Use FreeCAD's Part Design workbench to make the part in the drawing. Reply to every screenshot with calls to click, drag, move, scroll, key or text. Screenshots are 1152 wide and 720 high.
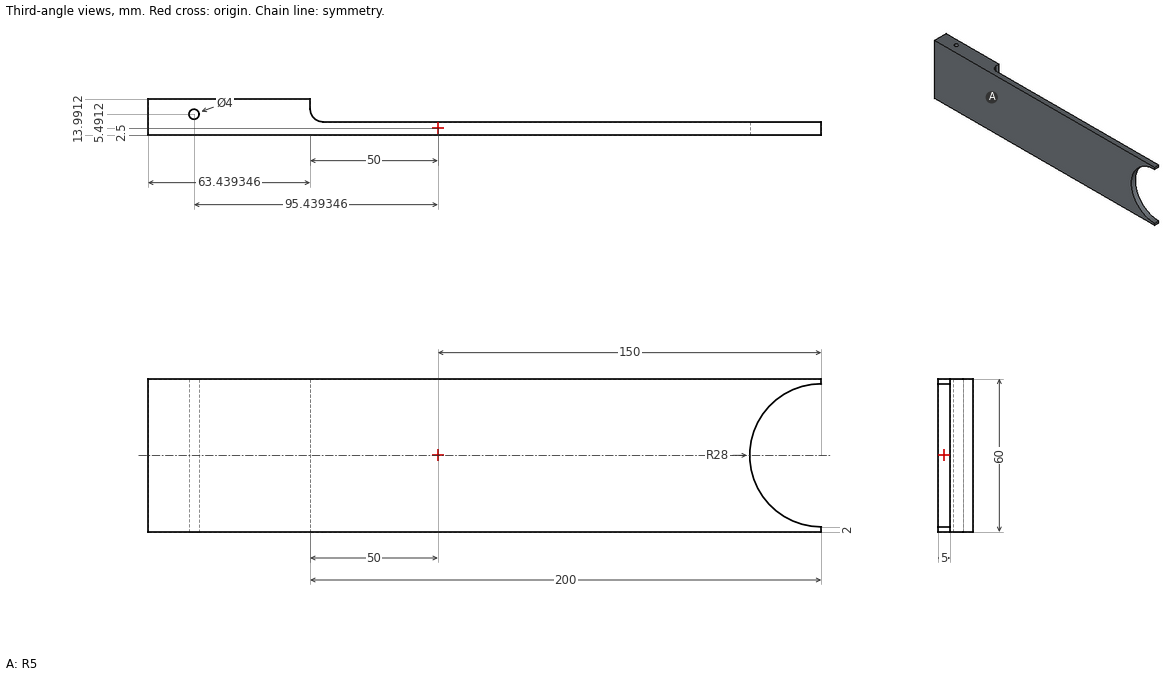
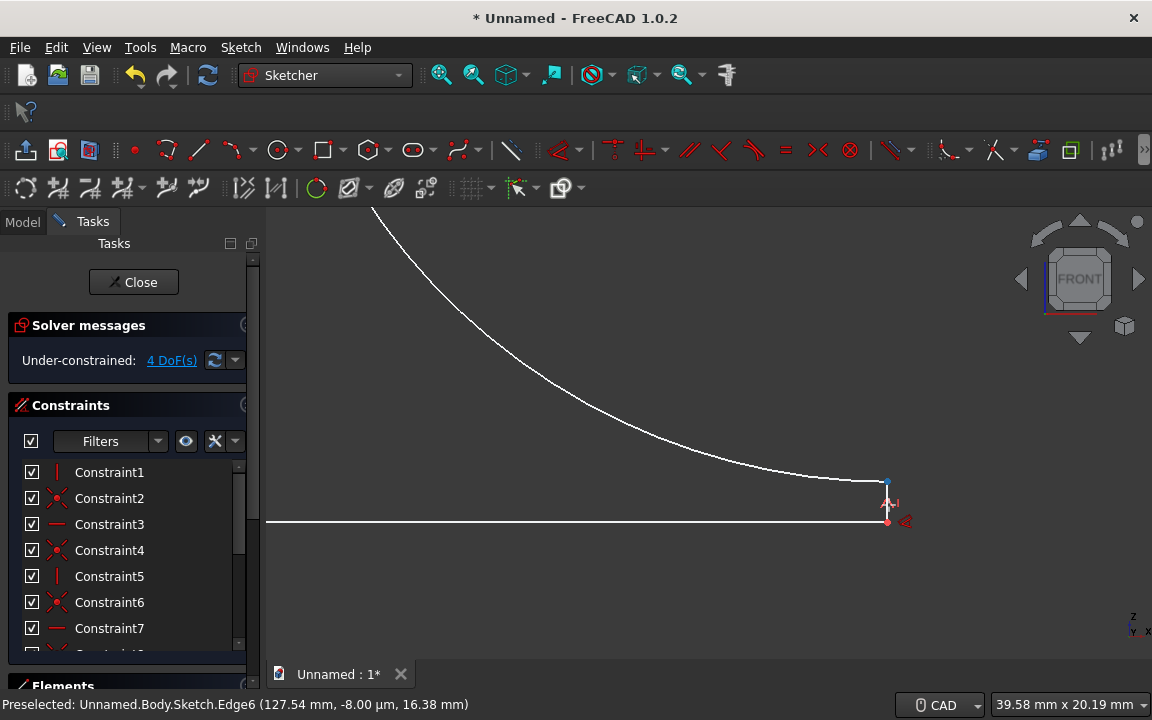
click(887, 502)
click(921, 502)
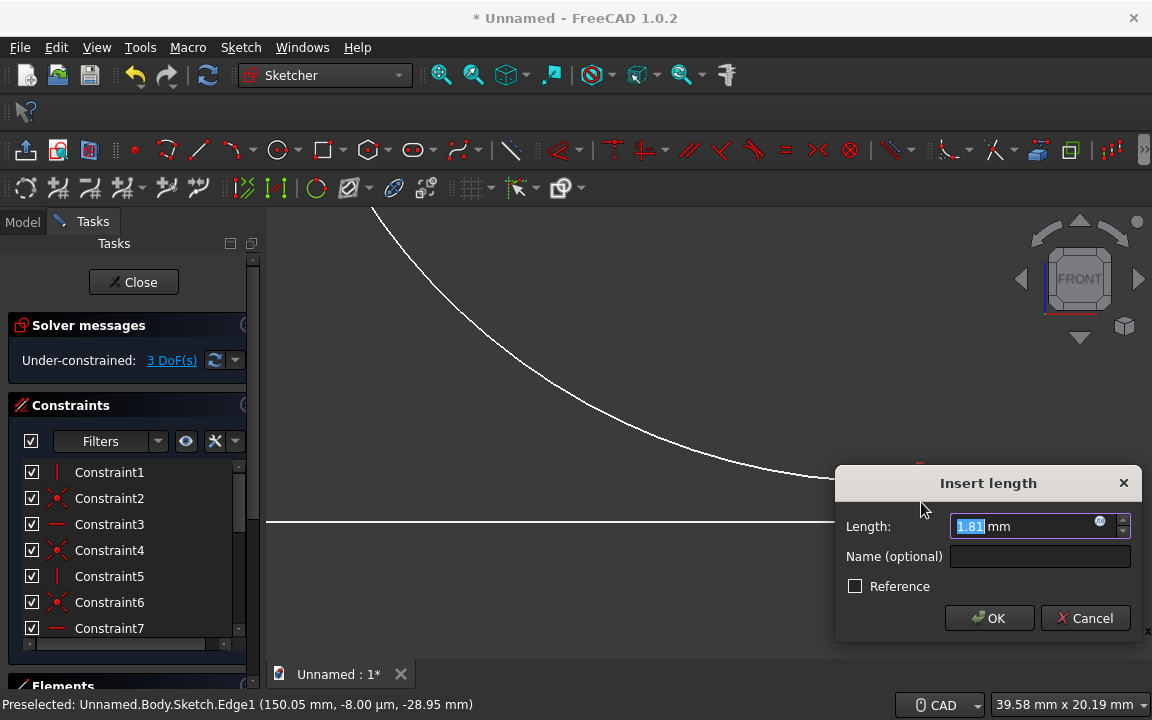
text(2)
key(Return)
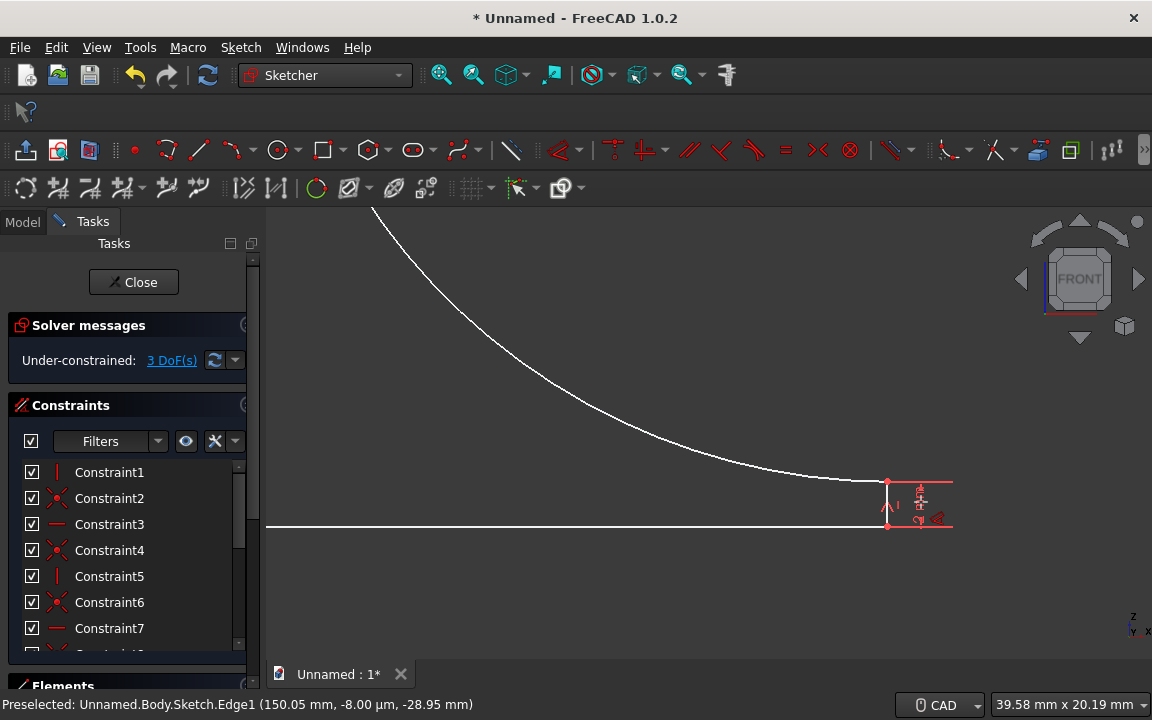
scroll(889, 505, down, 11)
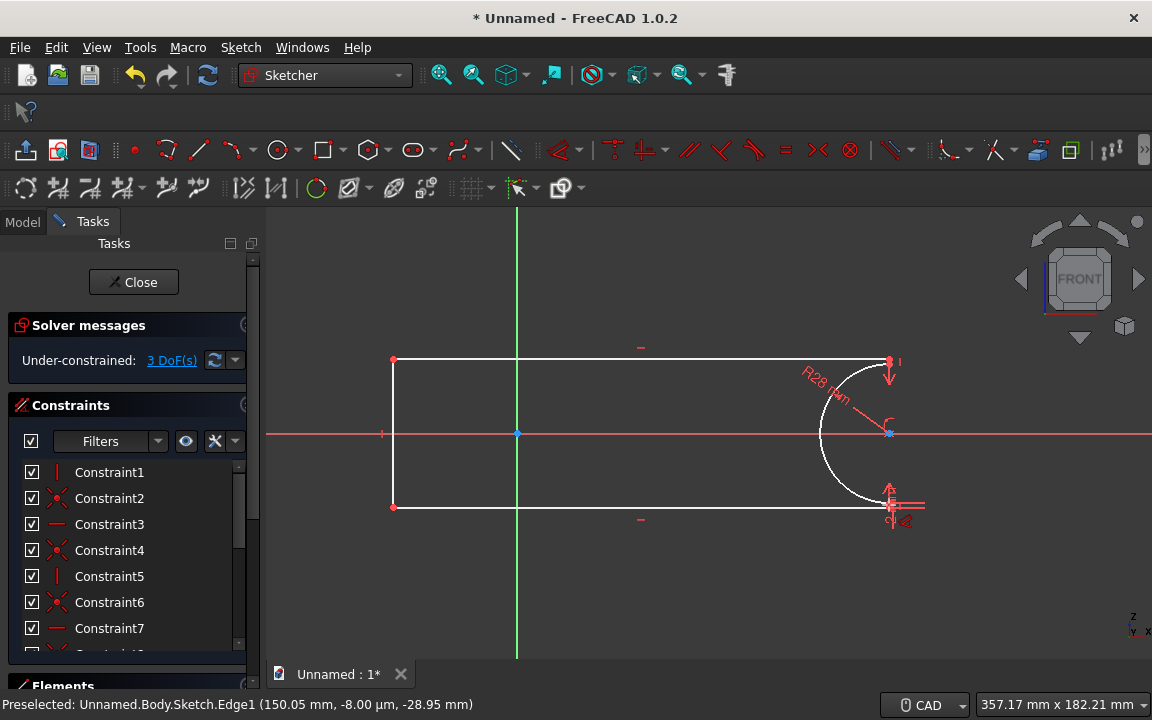
click(741, 508)
click(641, 542)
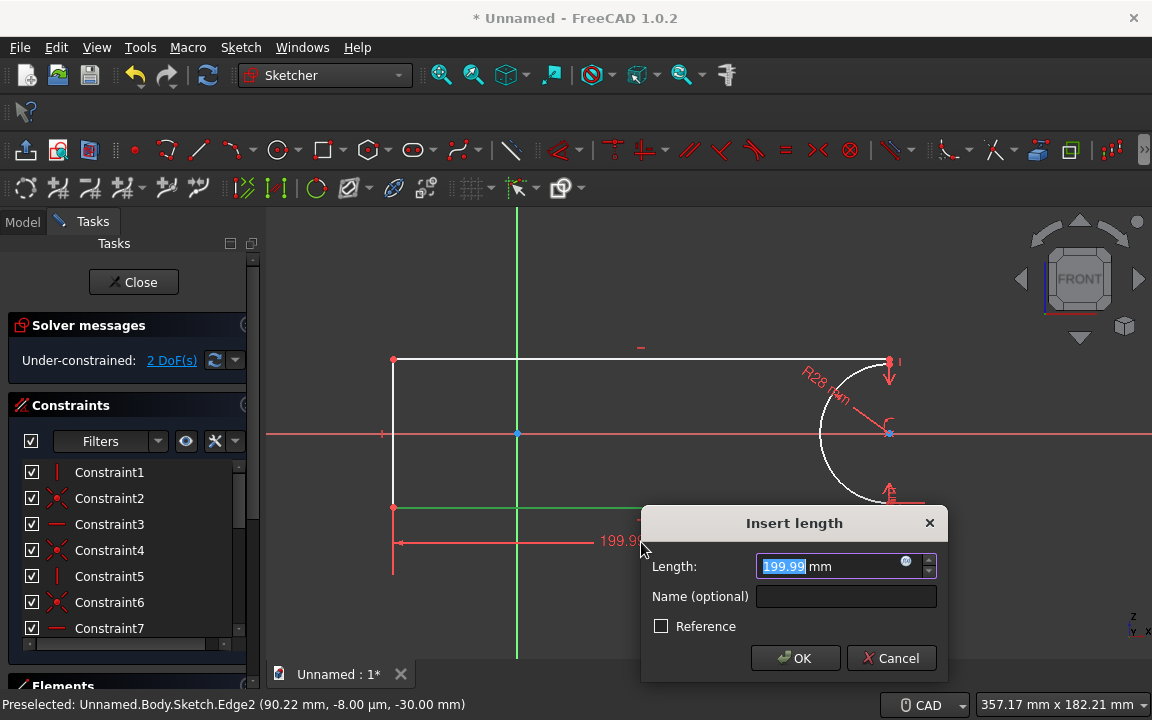
text(200)
key(Return)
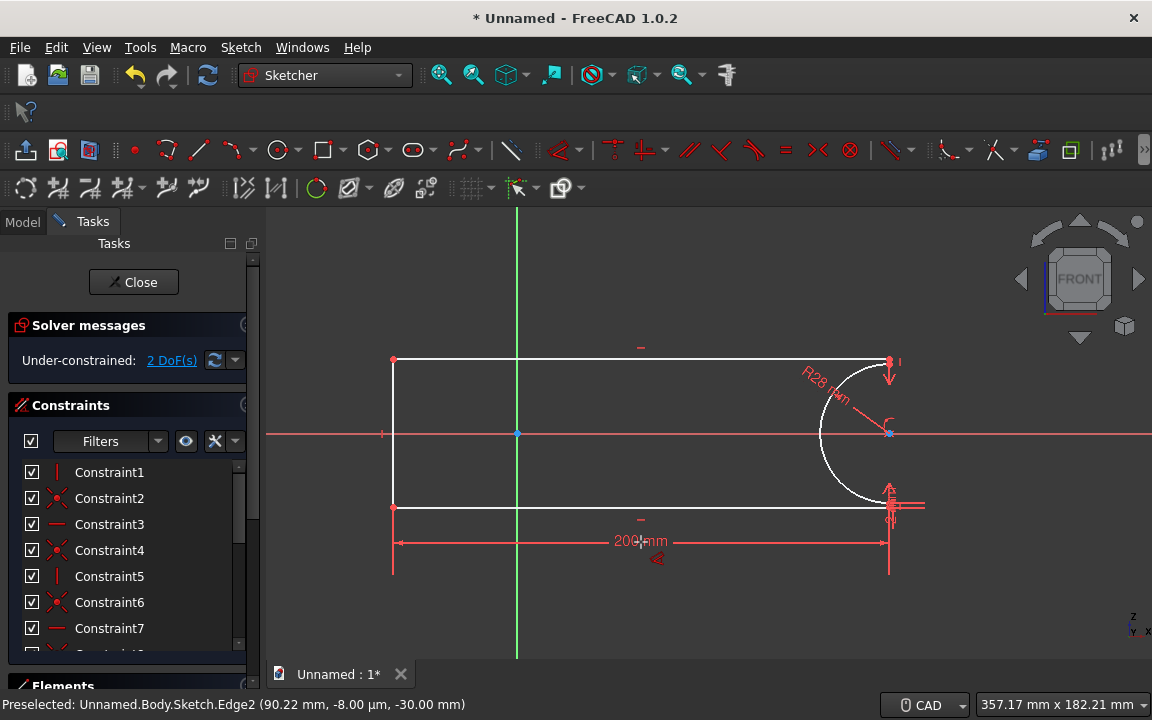
click(393, 508)
click(455, 542)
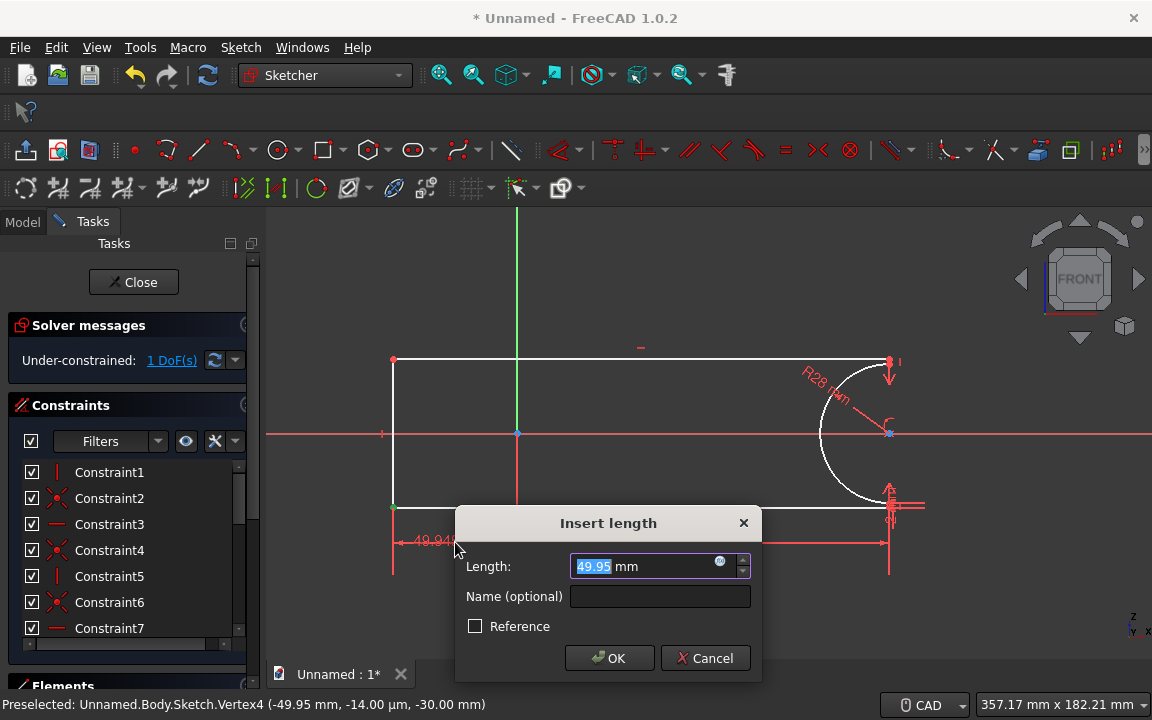
text(50)
key(Return)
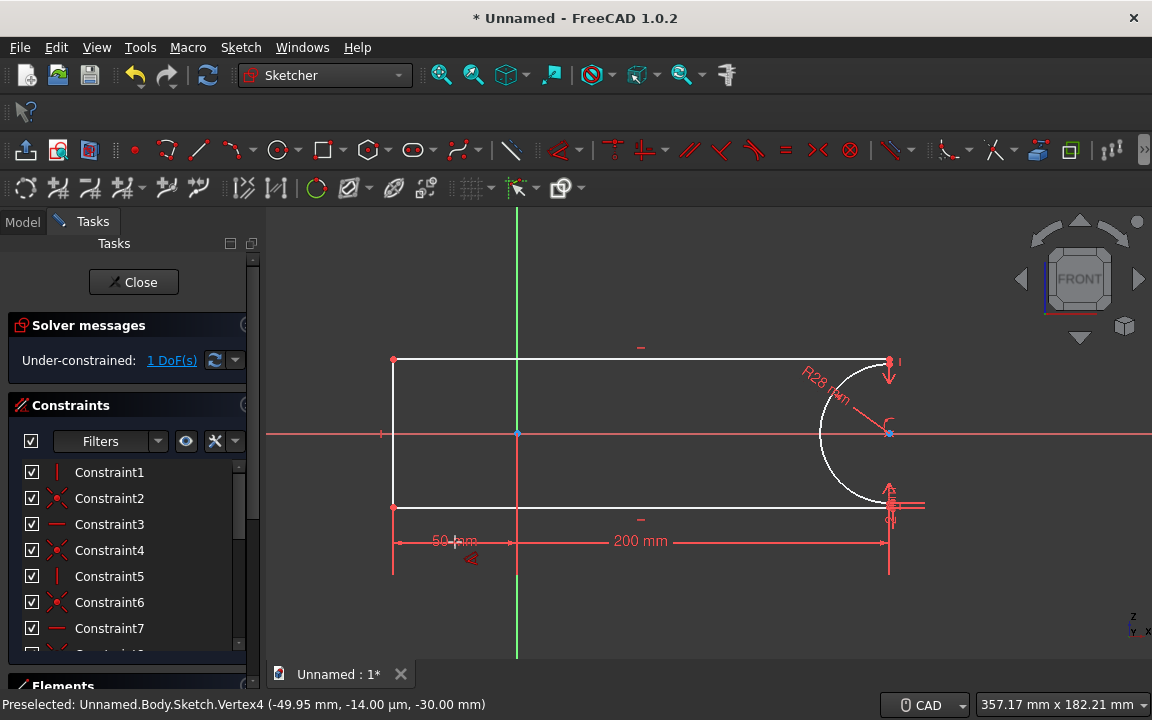
click(890, 434)
click(703, 468)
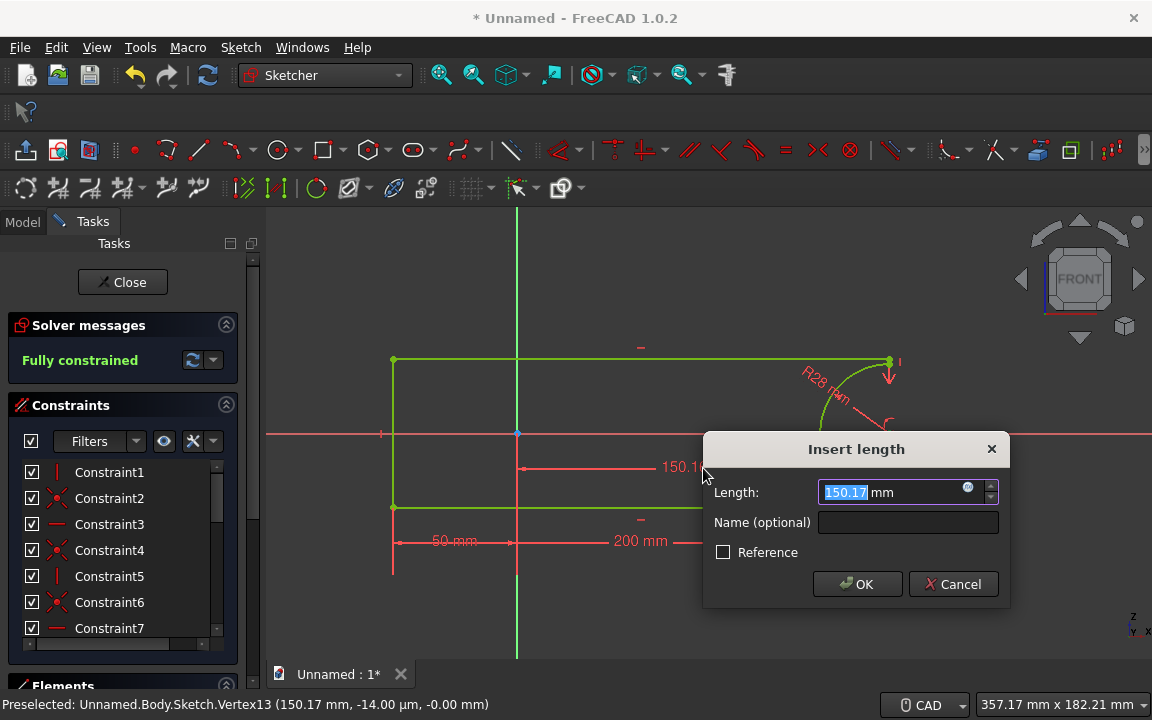
text(150)
key(Return)
key(Escape)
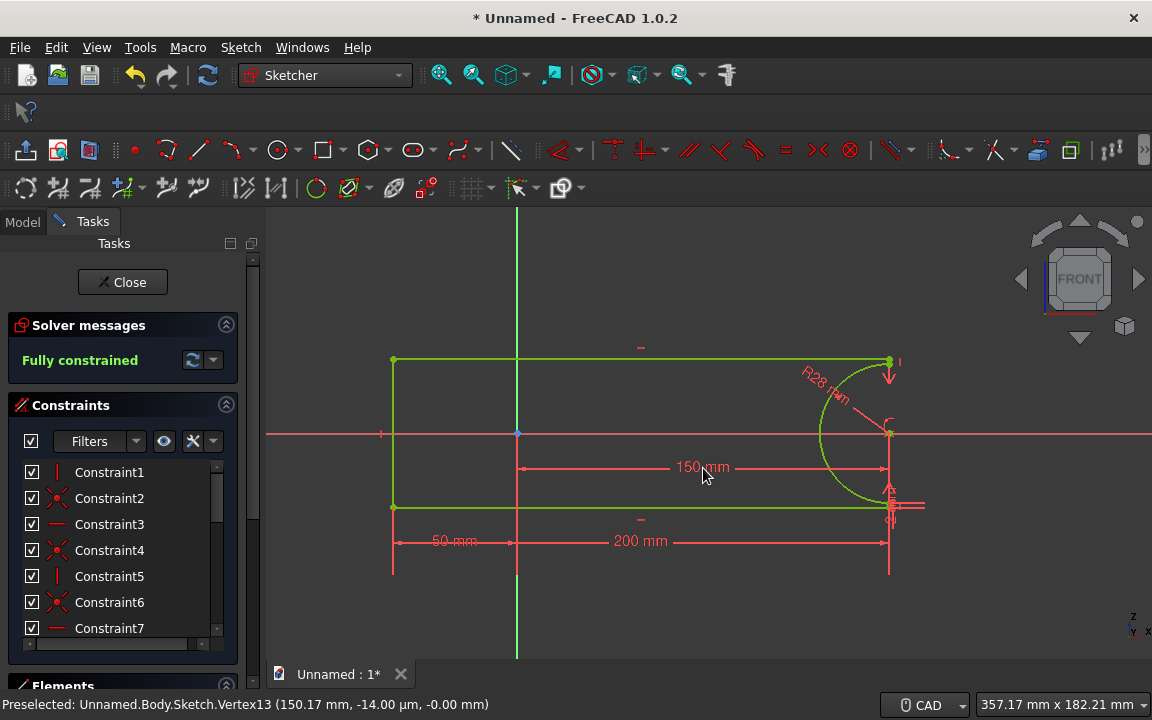
click(123, 282)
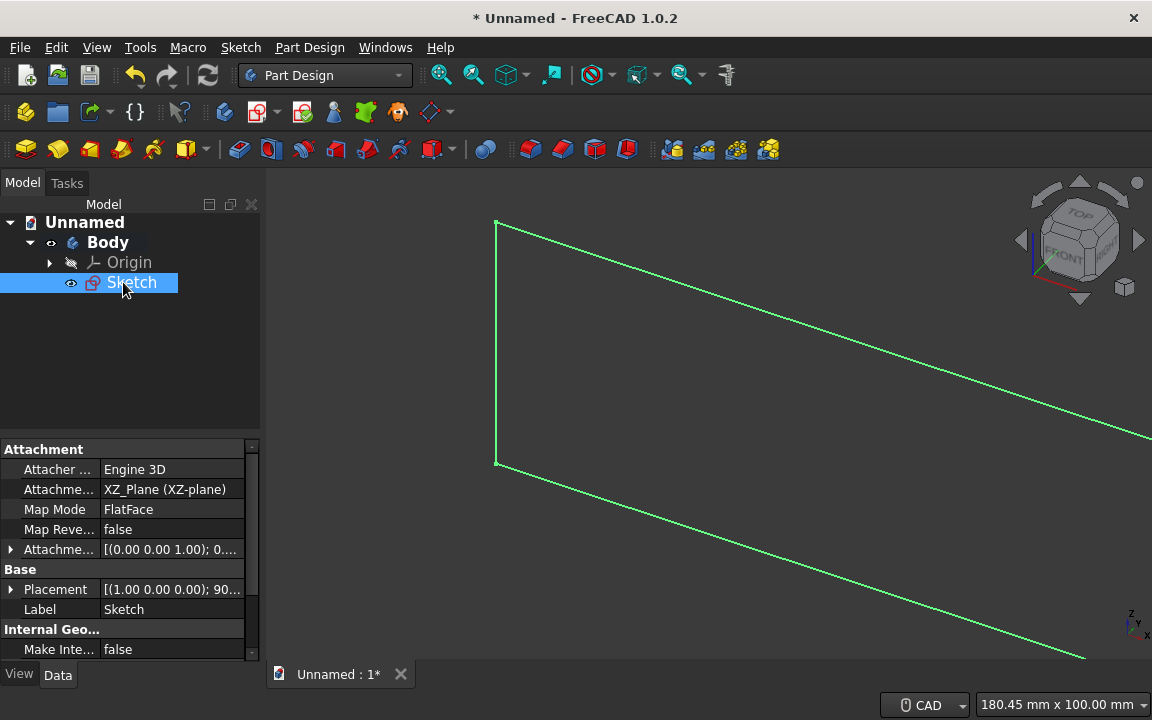
click(26, 150)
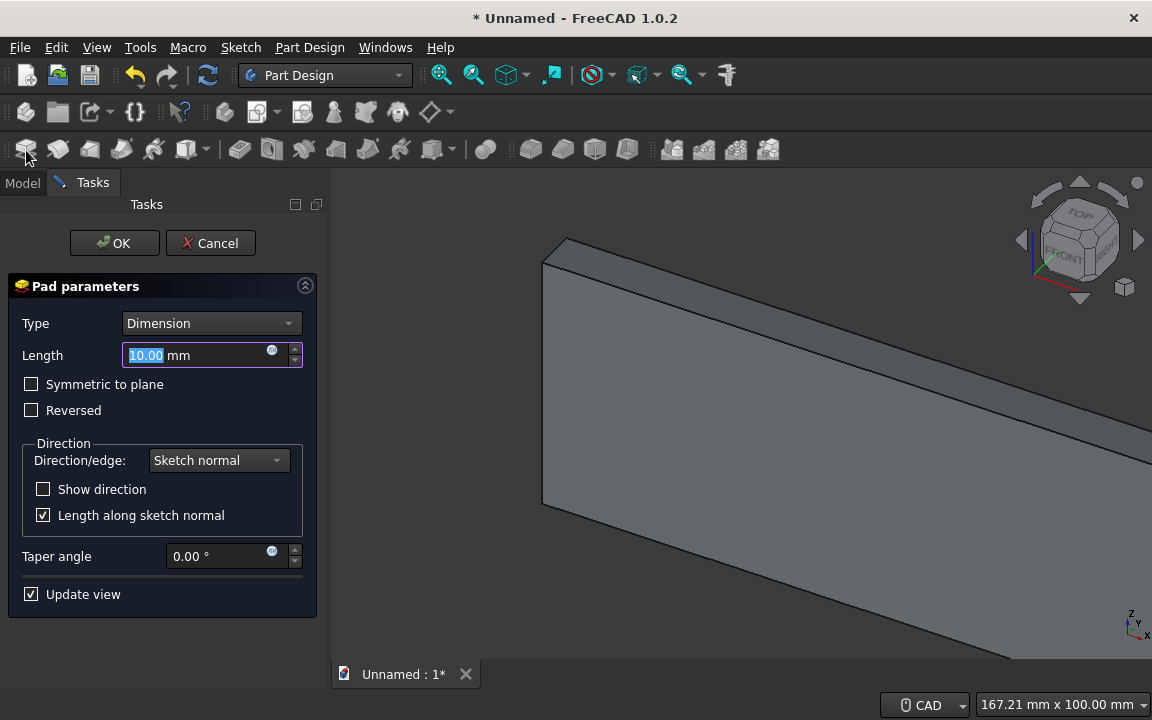
text(5)
key(Tab)